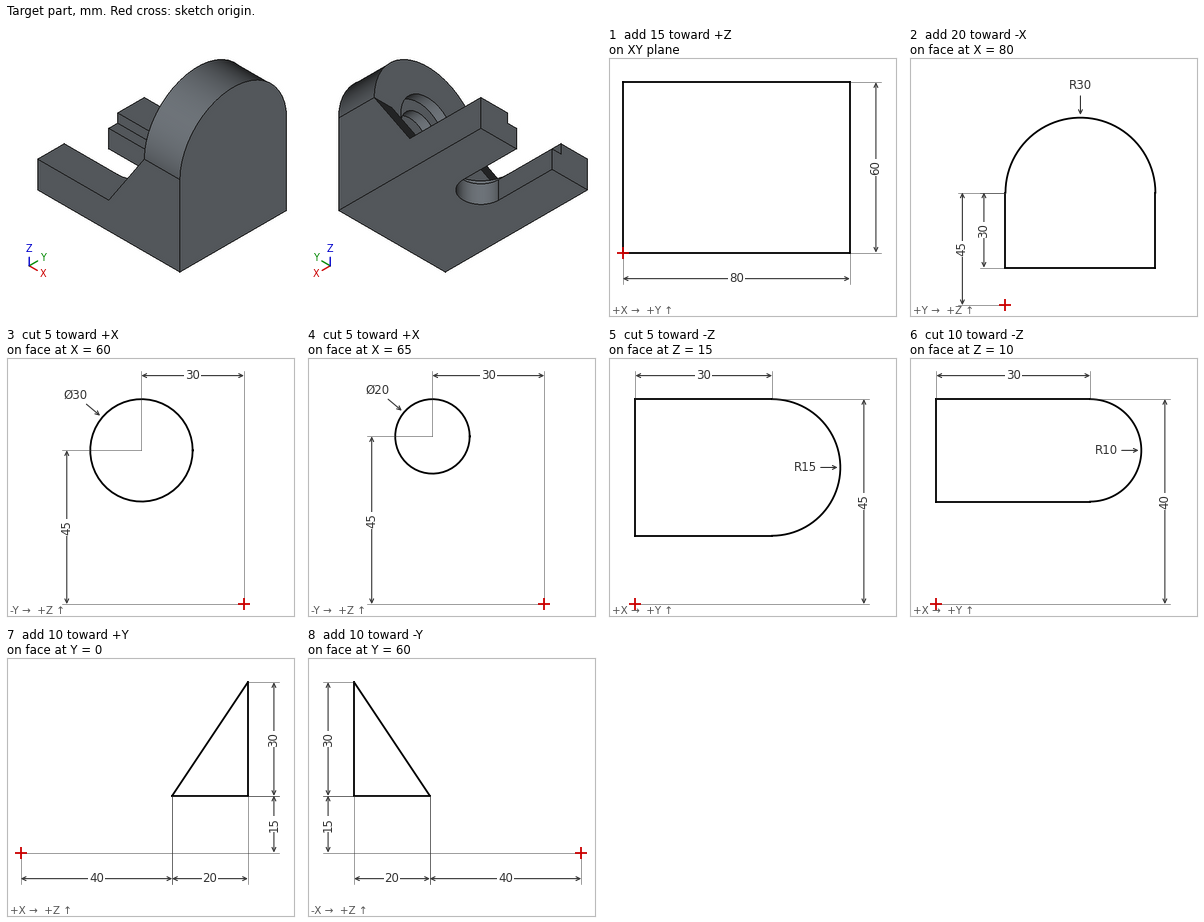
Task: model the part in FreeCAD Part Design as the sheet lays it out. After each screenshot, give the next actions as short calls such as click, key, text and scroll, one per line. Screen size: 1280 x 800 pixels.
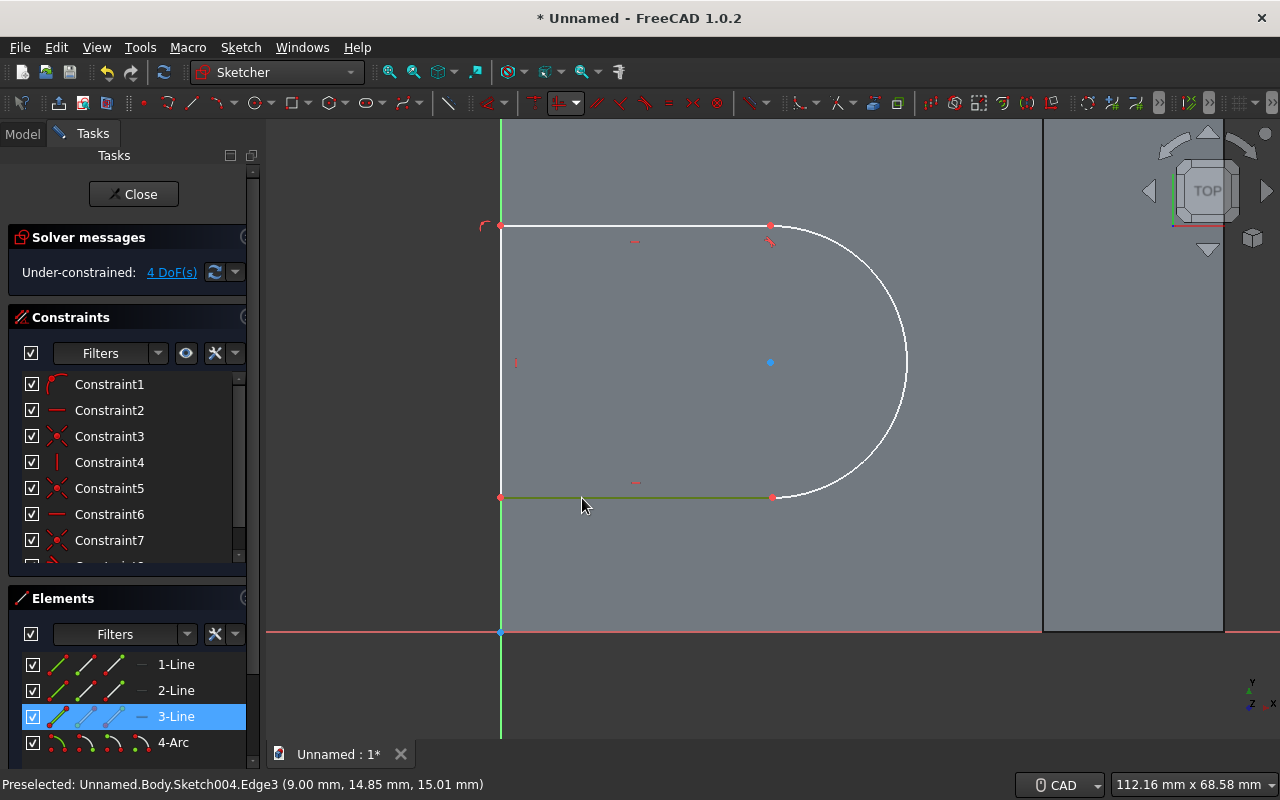
click(881, 441)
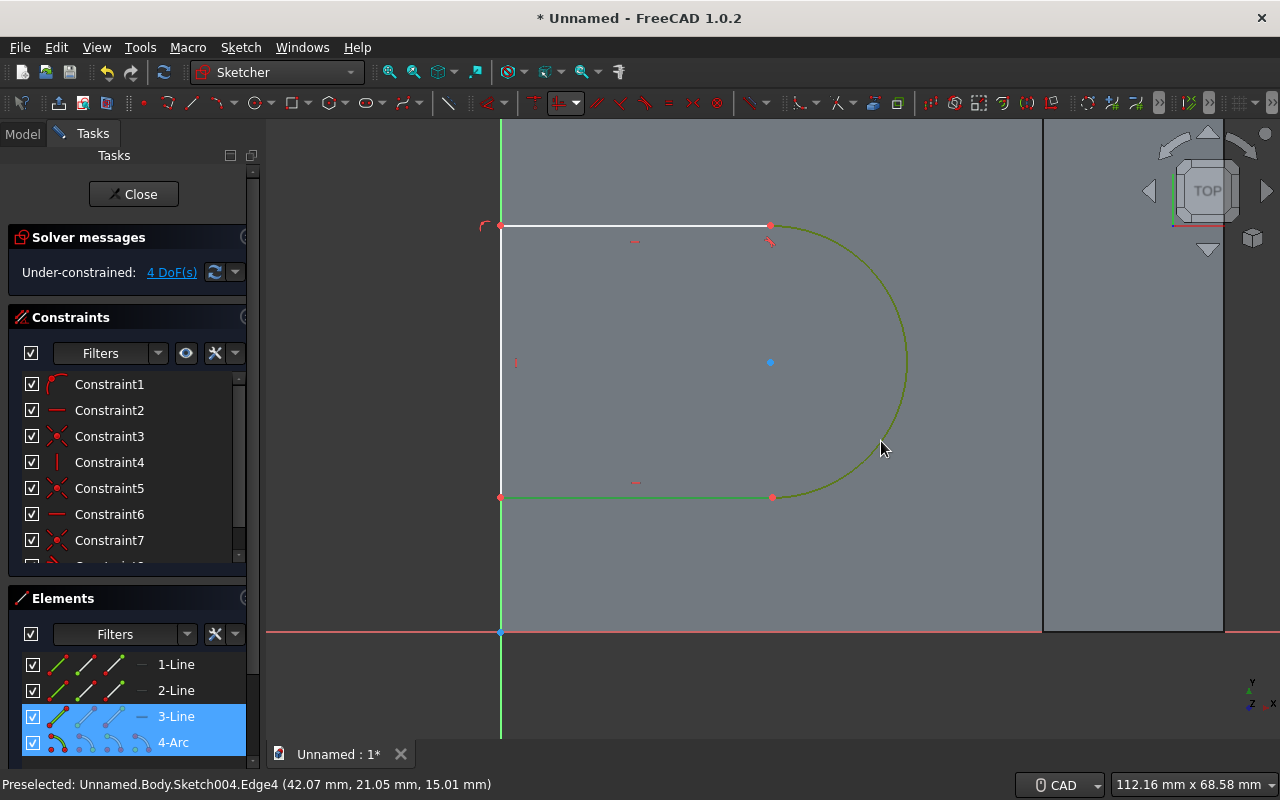
click(646, 104)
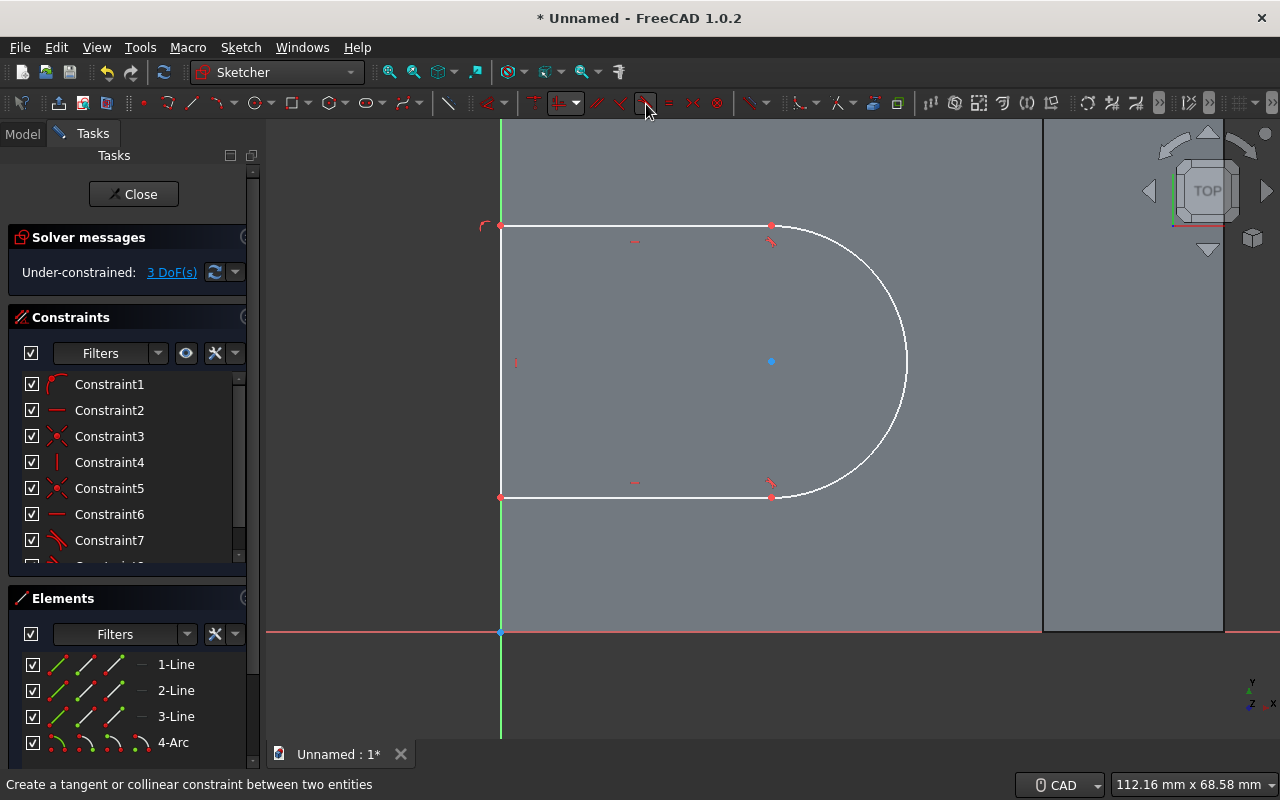
click(488, 104)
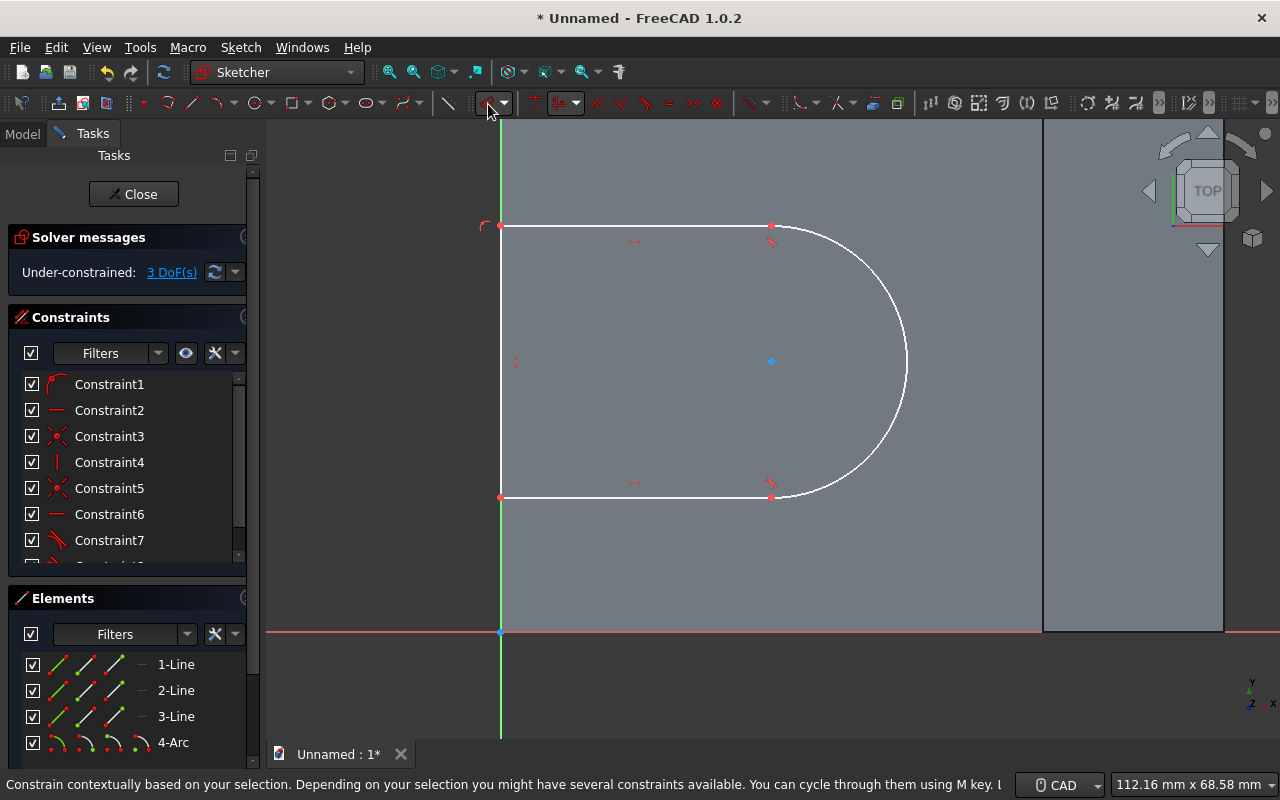
click(881, 442)
click(907, 461)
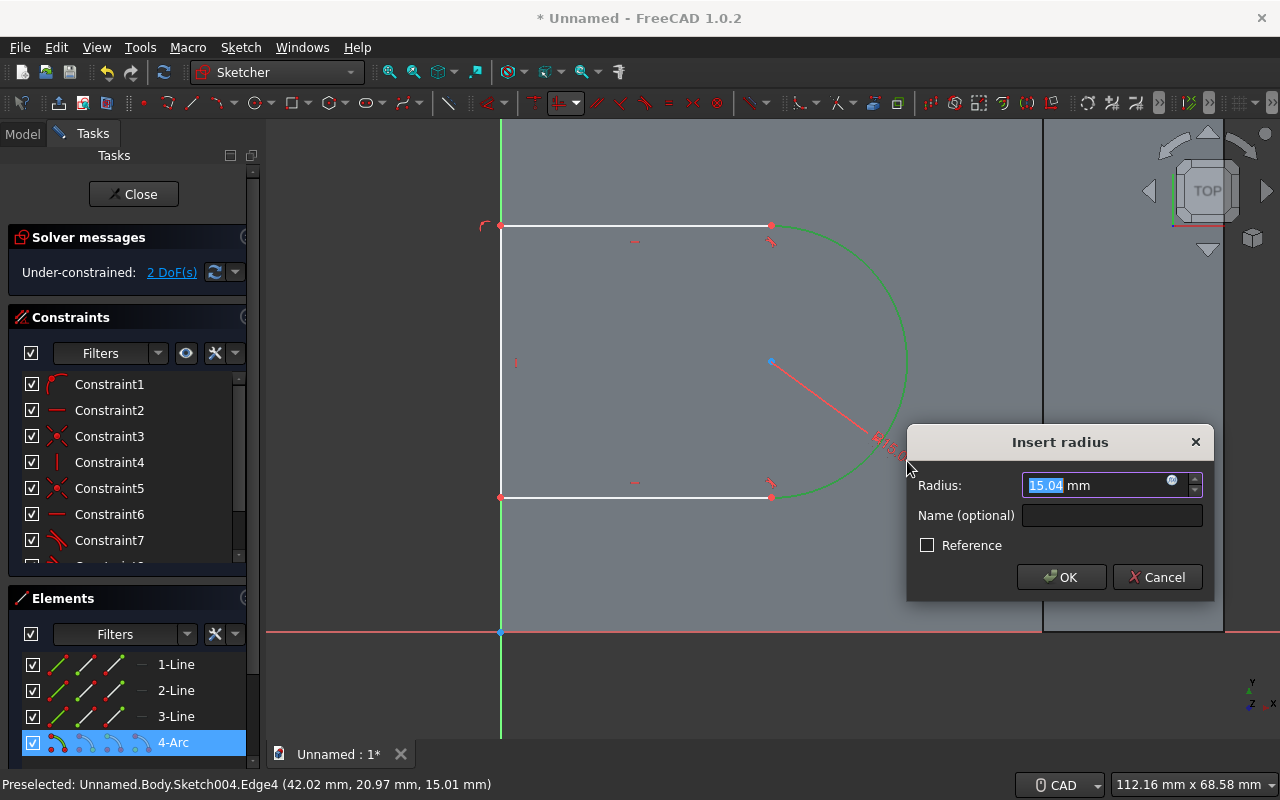
text(15)
key(Return)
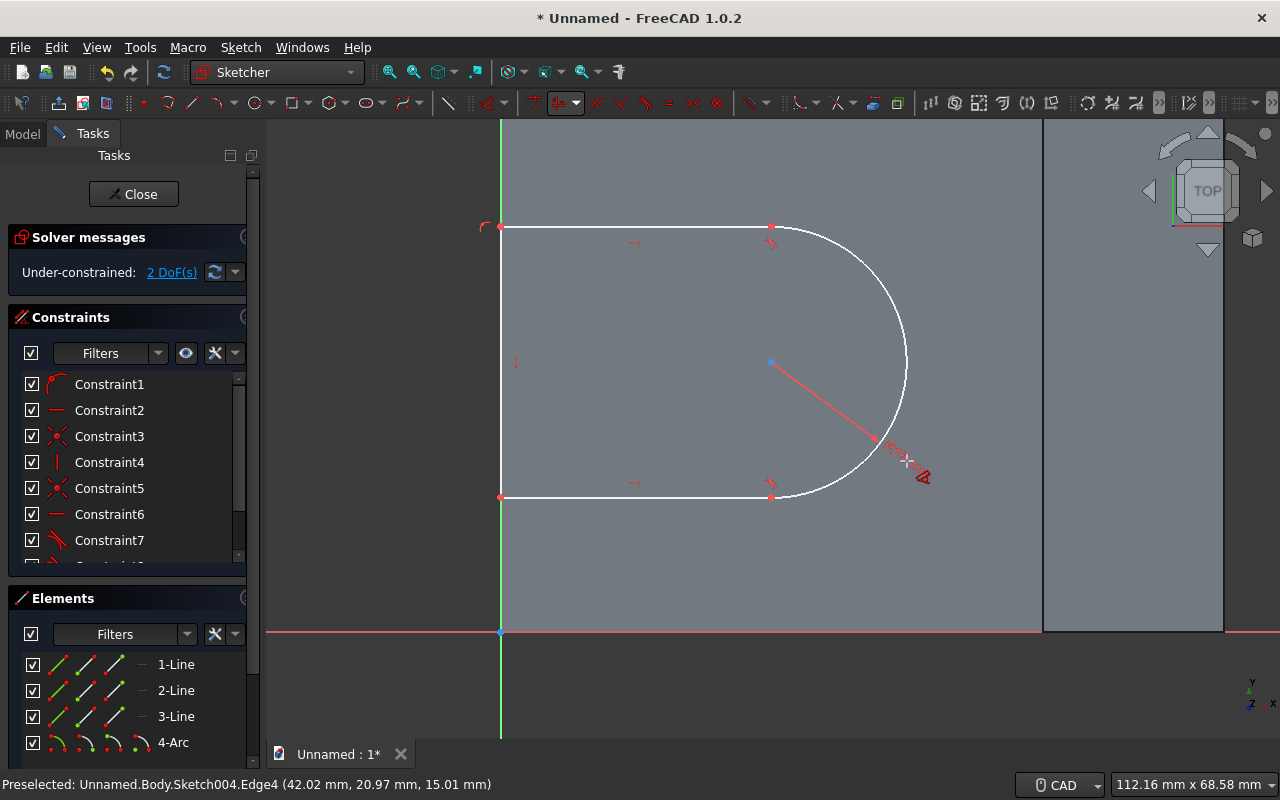
click(690, 227)
click(636, 193)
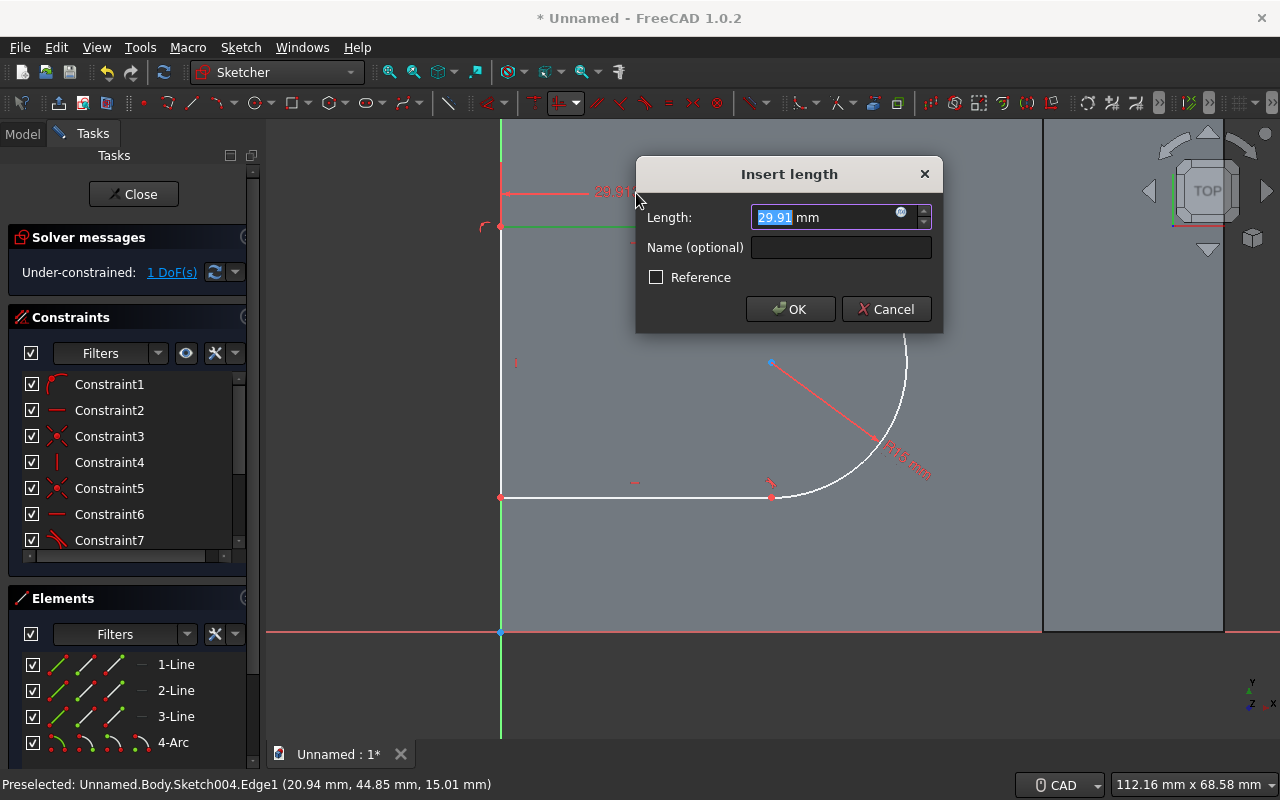
text(30)
key(Return)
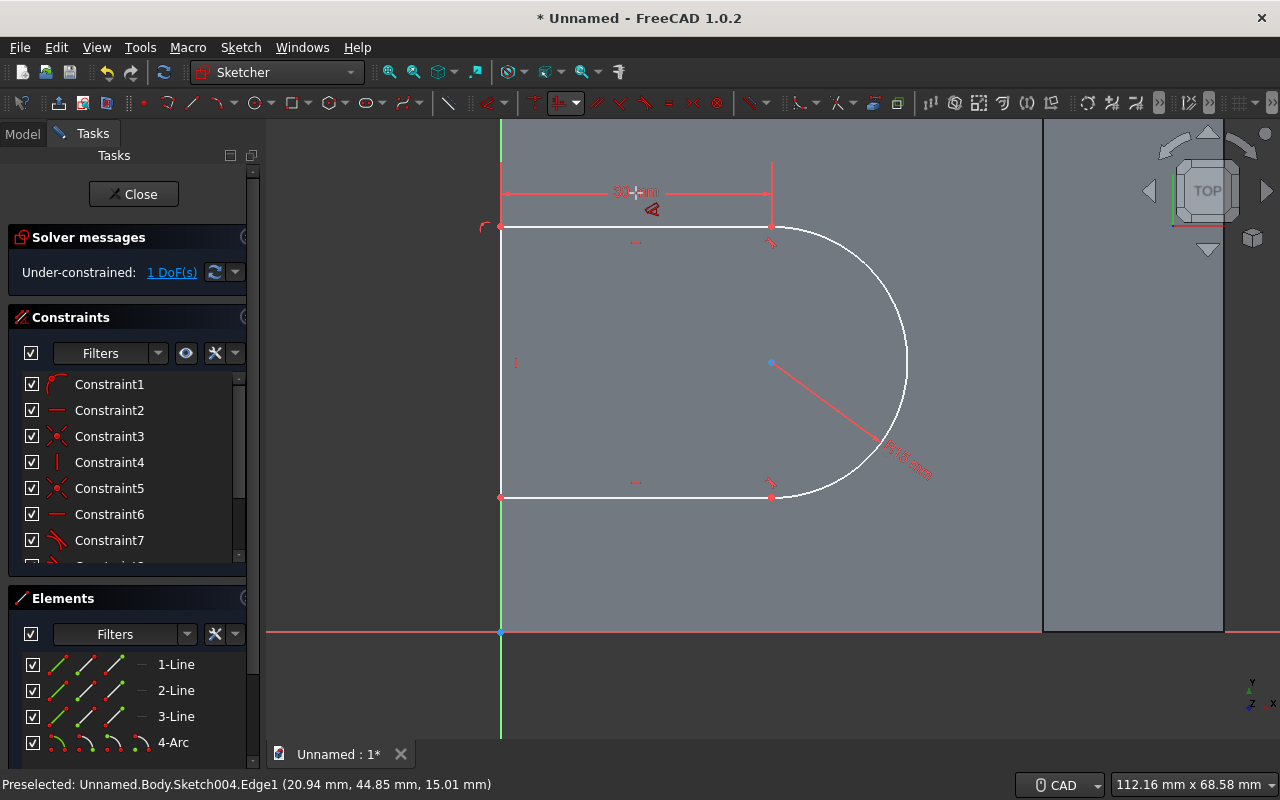
click(772, 227)
click(467, 430)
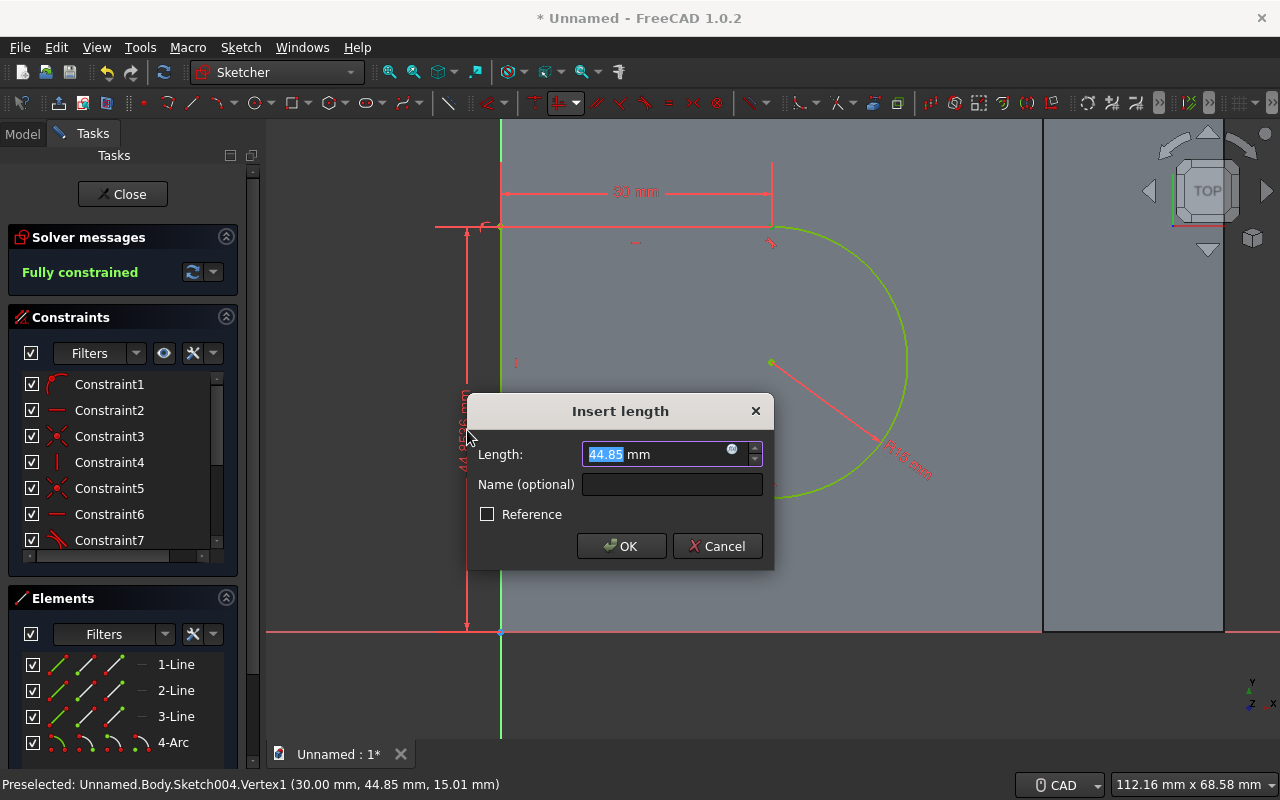
text(45)
key(Return)
key(Escape)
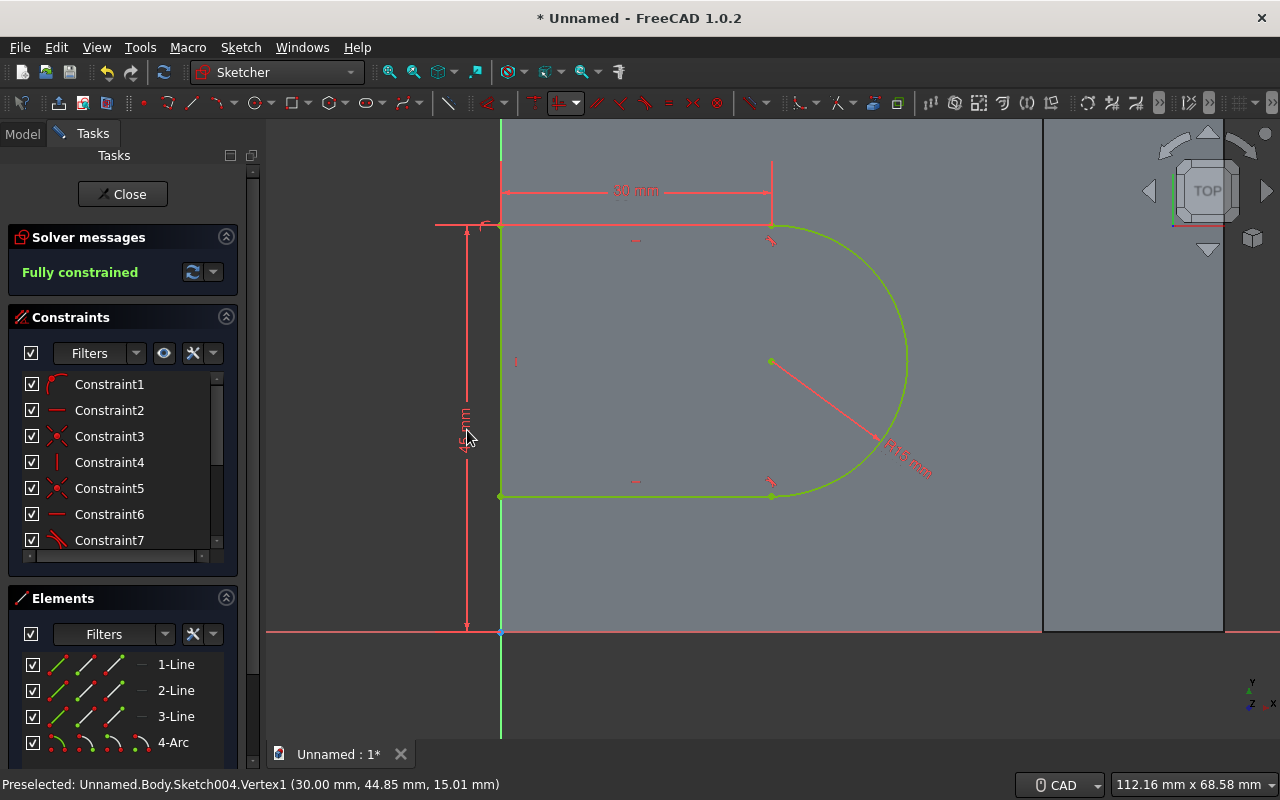
click(123, 194)